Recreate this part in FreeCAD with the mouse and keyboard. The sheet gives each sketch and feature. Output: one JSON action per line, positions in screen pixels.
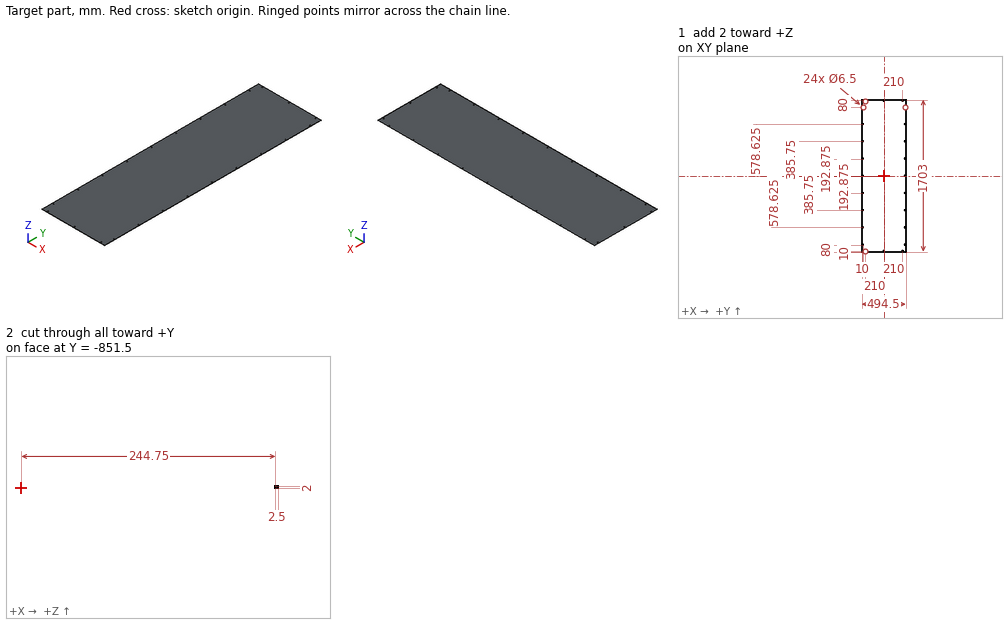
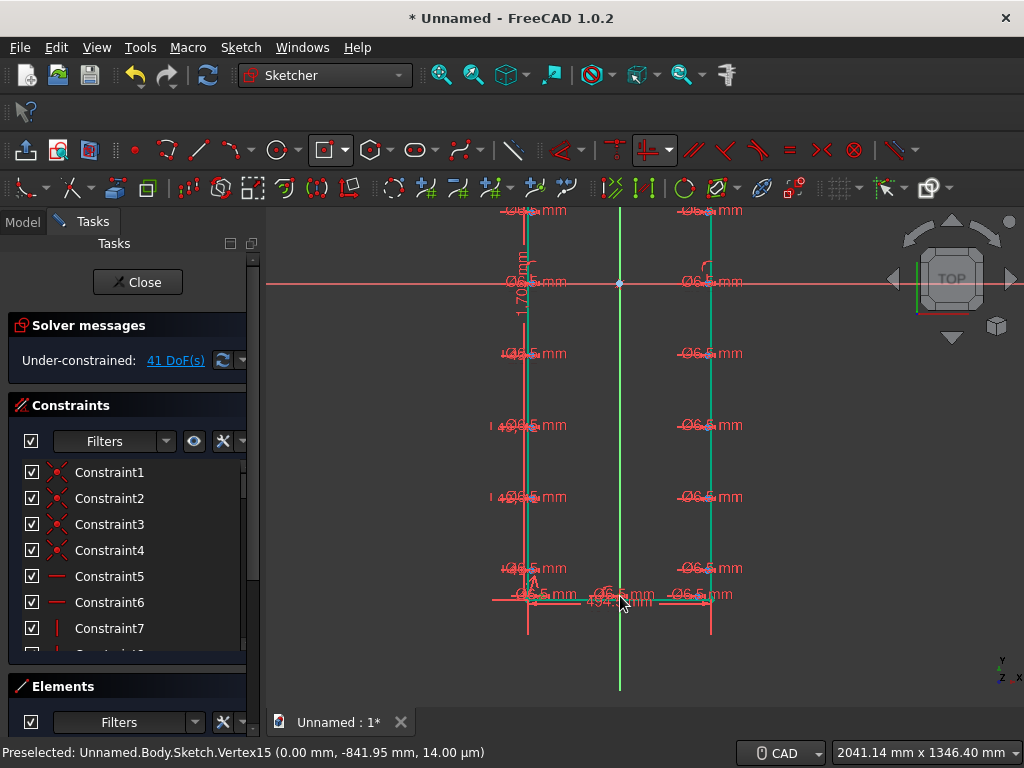
{"action": "left_click", "coordinate": [672, 150]}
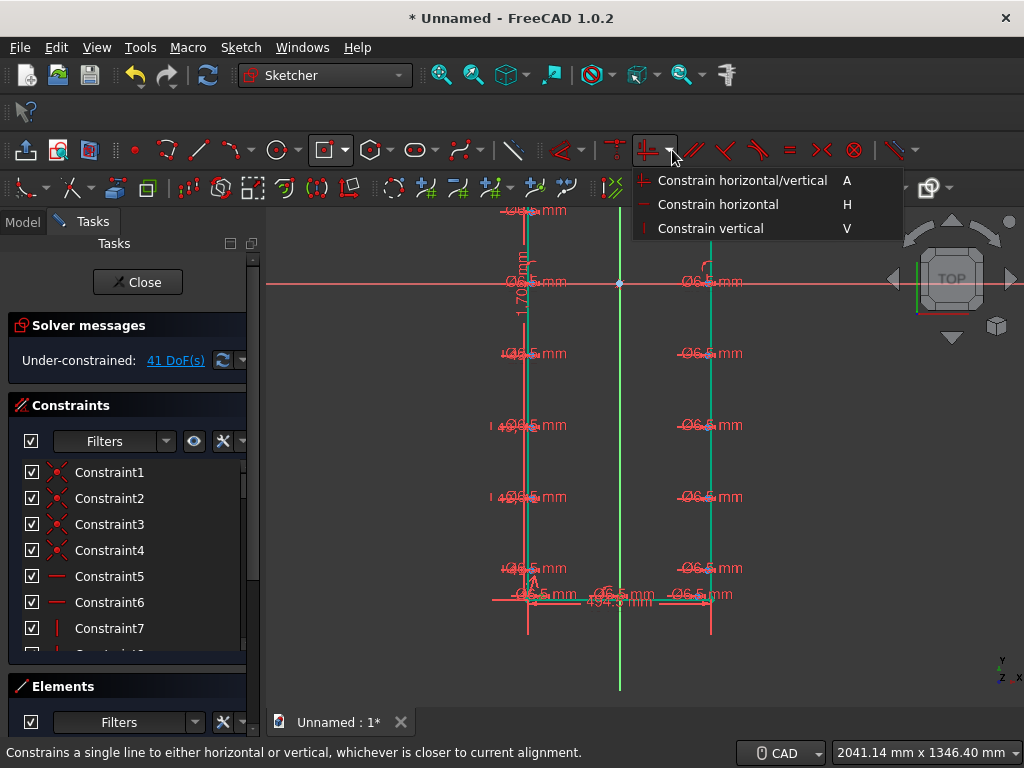
{"action": "left_click", "coordinate": [768, 204]}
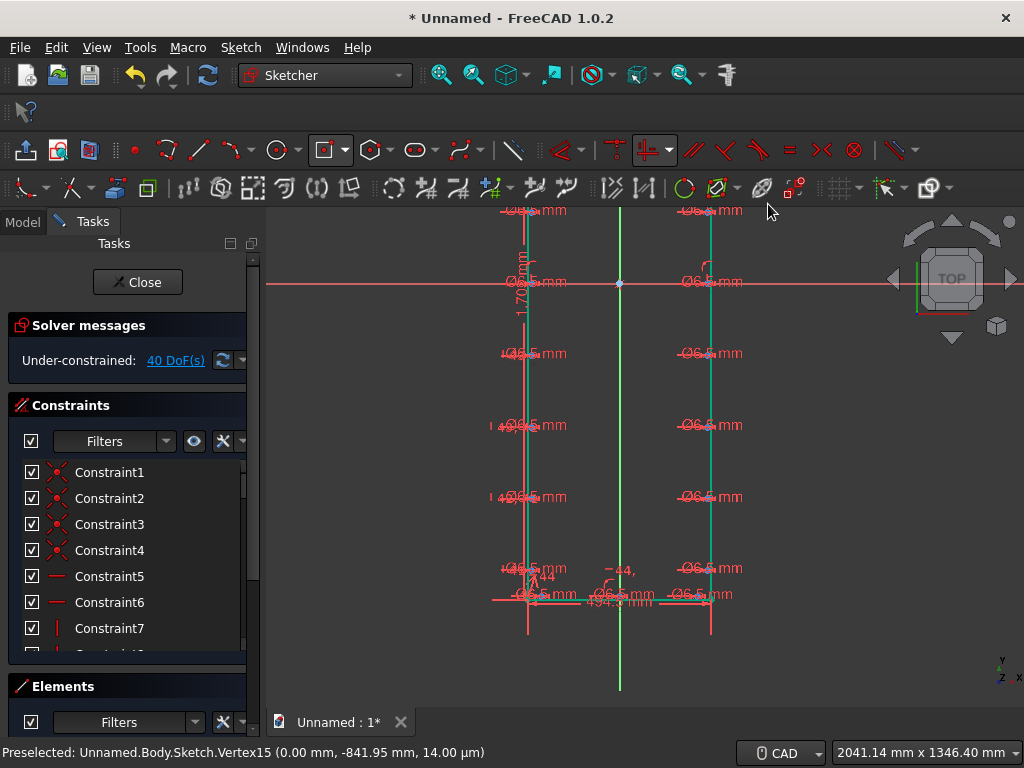
{"action": "left_click", "coordinate": [620, 596]}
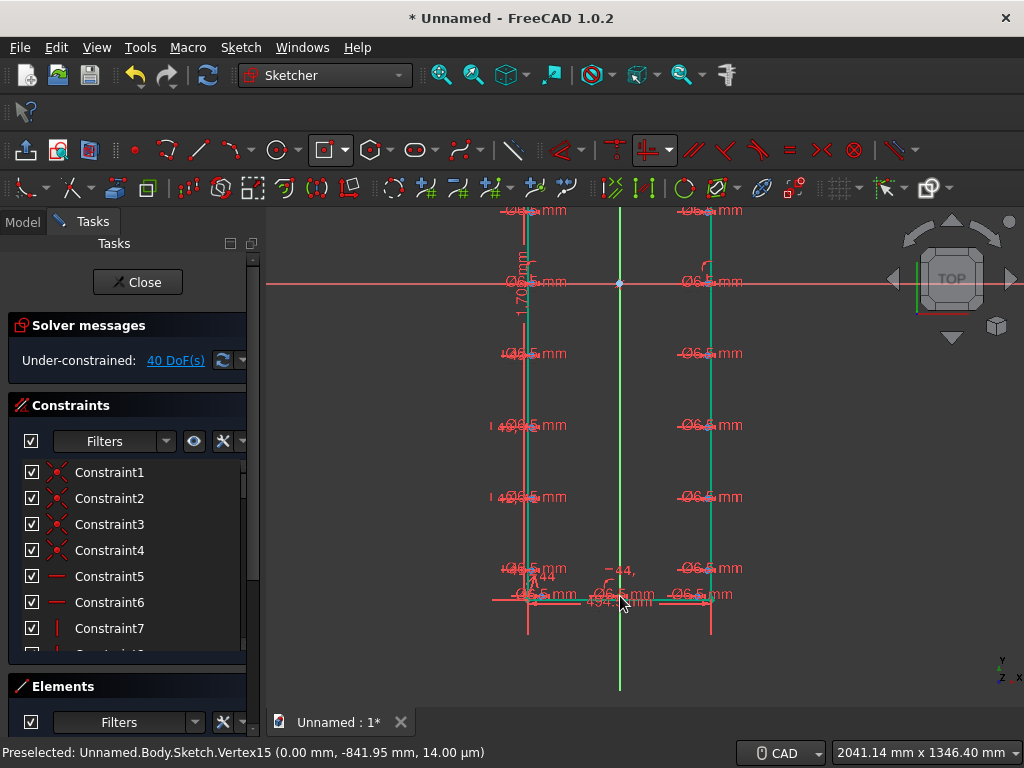
{"action": "left_click", "coordinate": [698, 596]}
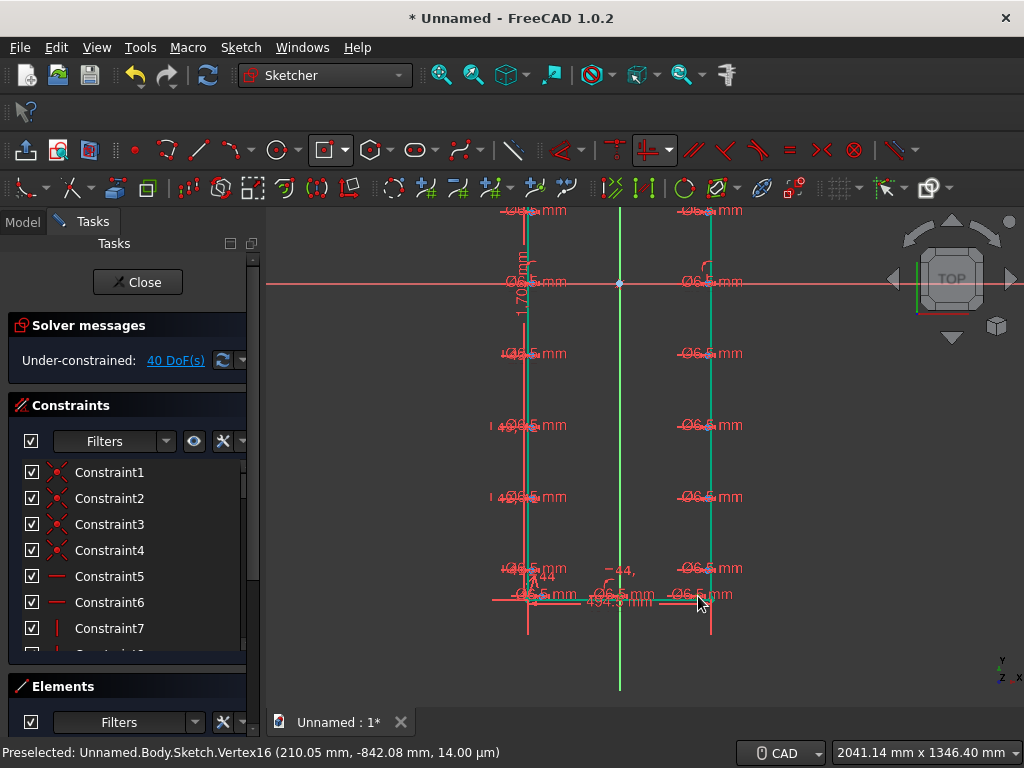
{"action": "left_click", "coordinate": [672, 150]}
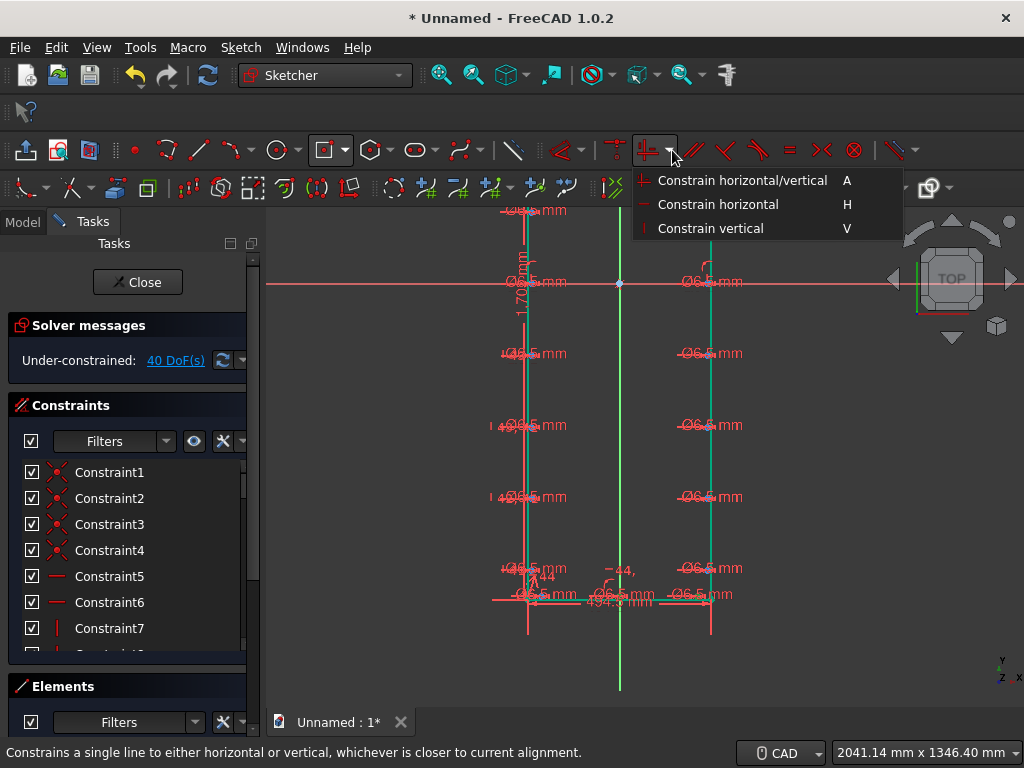
{"action": "left_click", "coordinate": [768, 204]}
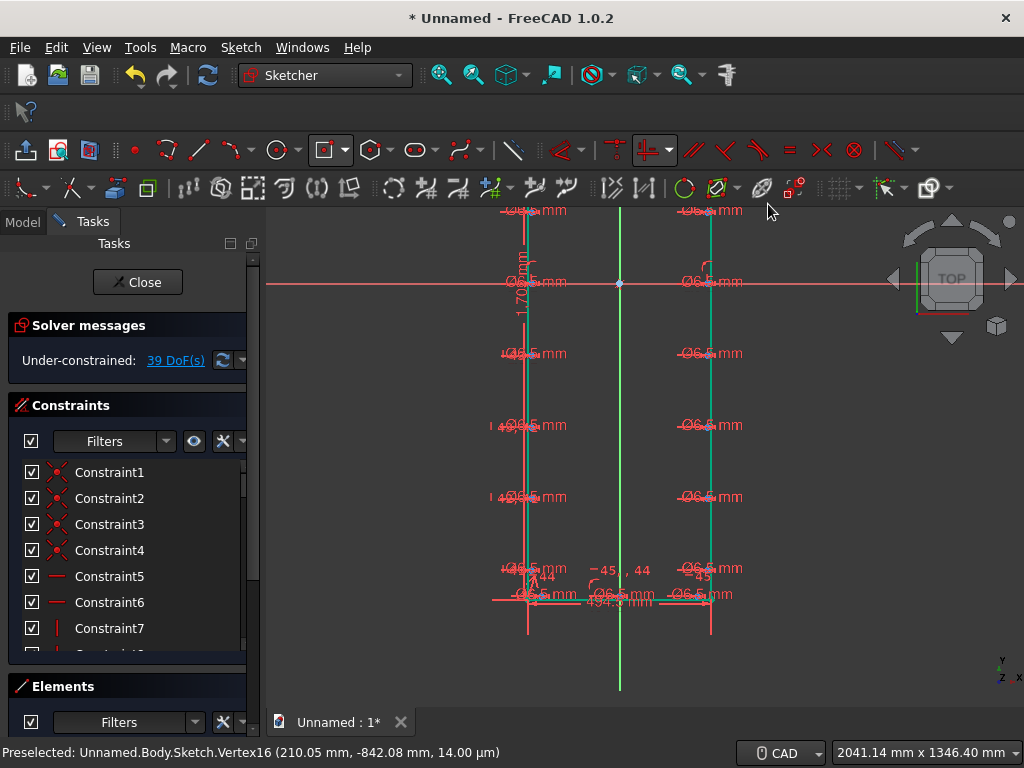
{"action": "left_click", "coordinate": [532, 570]}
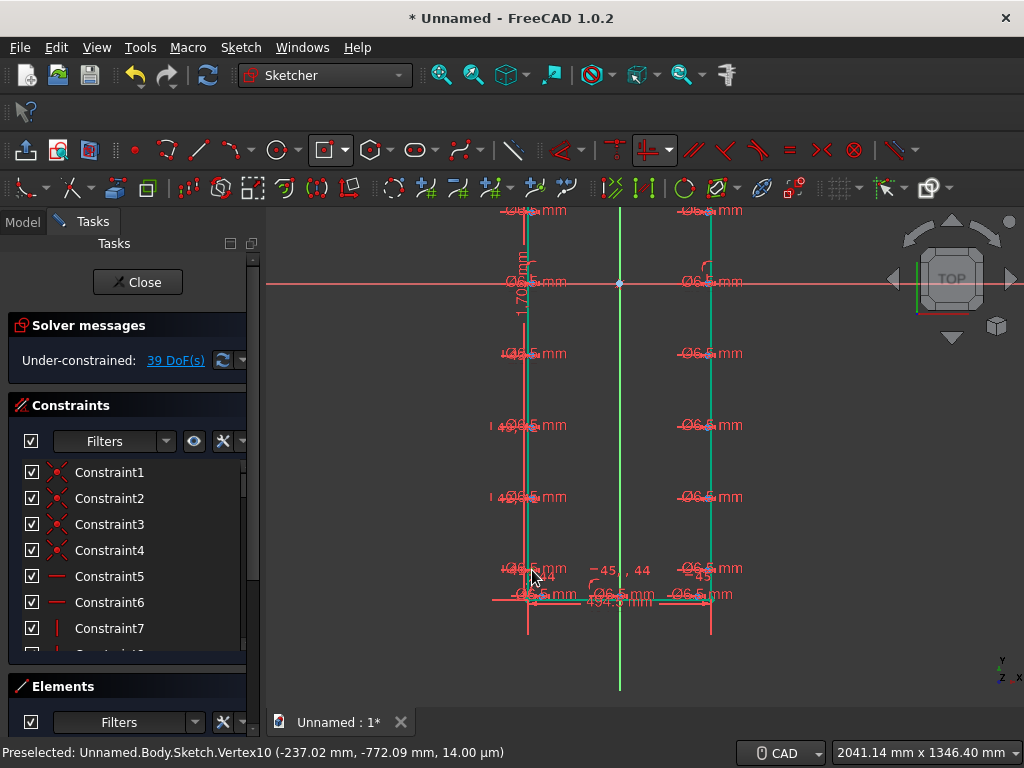
{"action": "scroll", "coordinate": [708, 570], "scroll_direction": "up", "scroll_amount": 4}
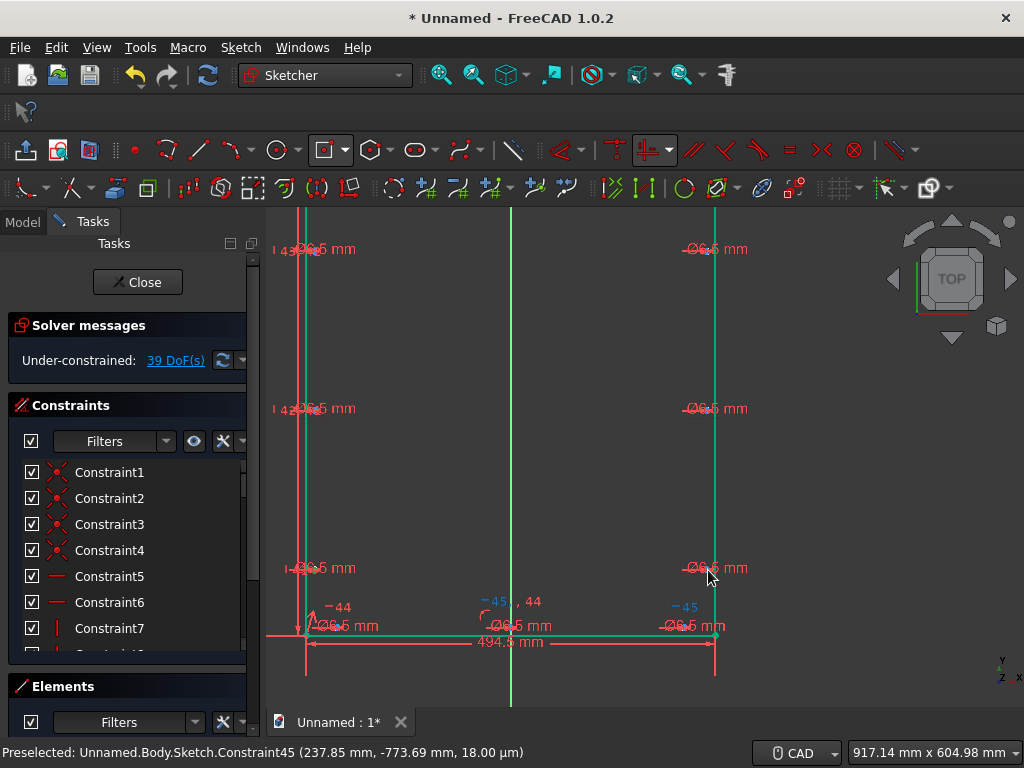
{"action": "left_click", "coordinate": [707, 570]}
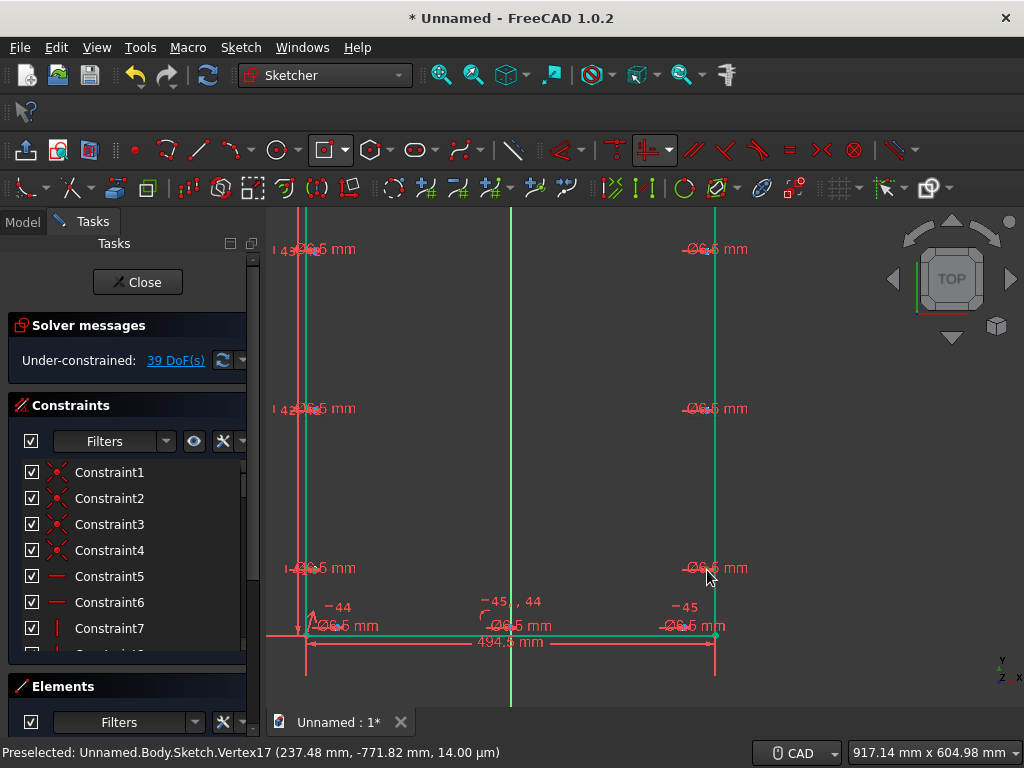
{"action": "key", "text": "h"}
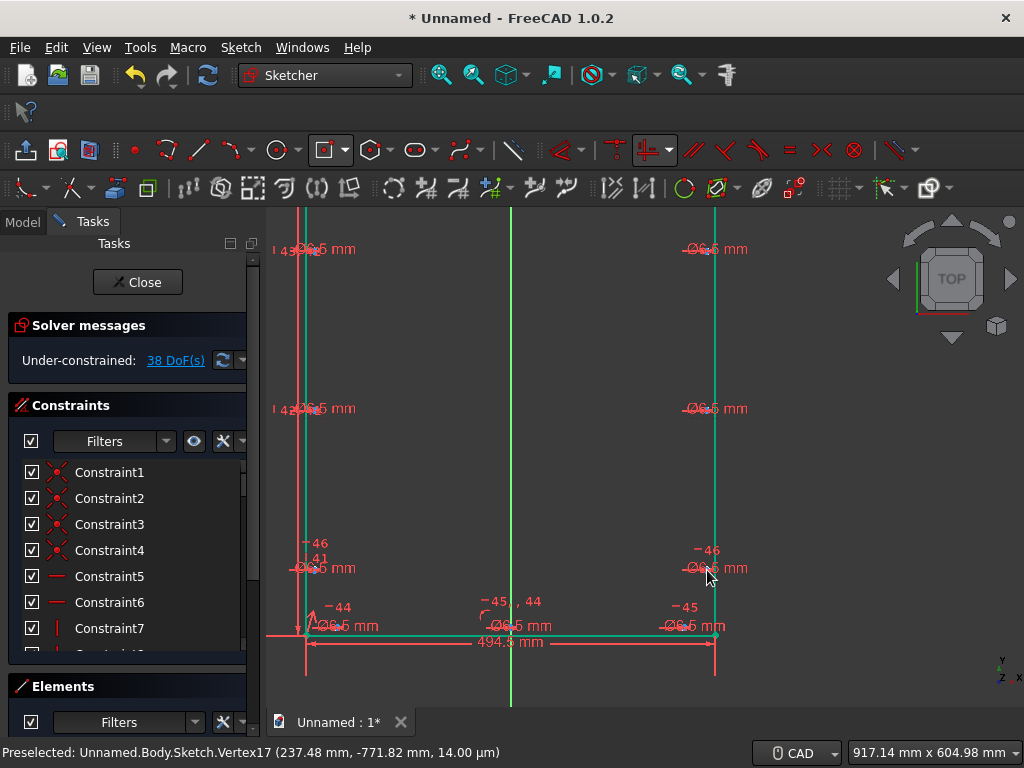
{"action": "scroll", "coordinate": [593, 590], "scroll_direction": "down", "scroll_amount": 8}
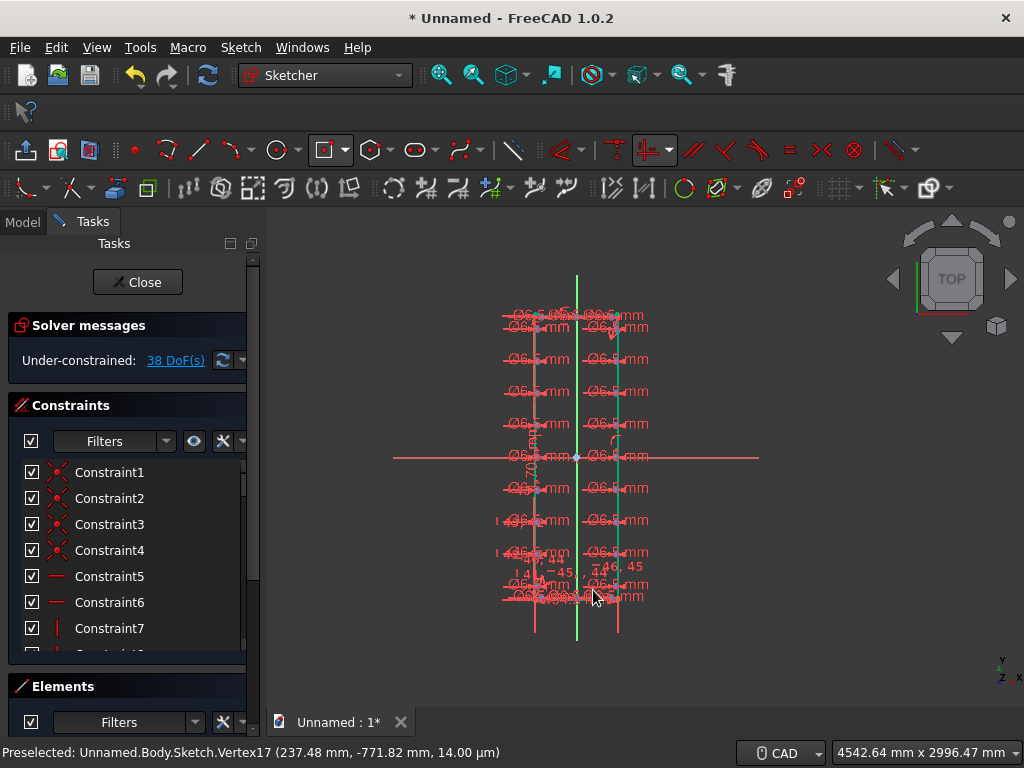
{"action": "left_click", "coordinate": [616, 587]}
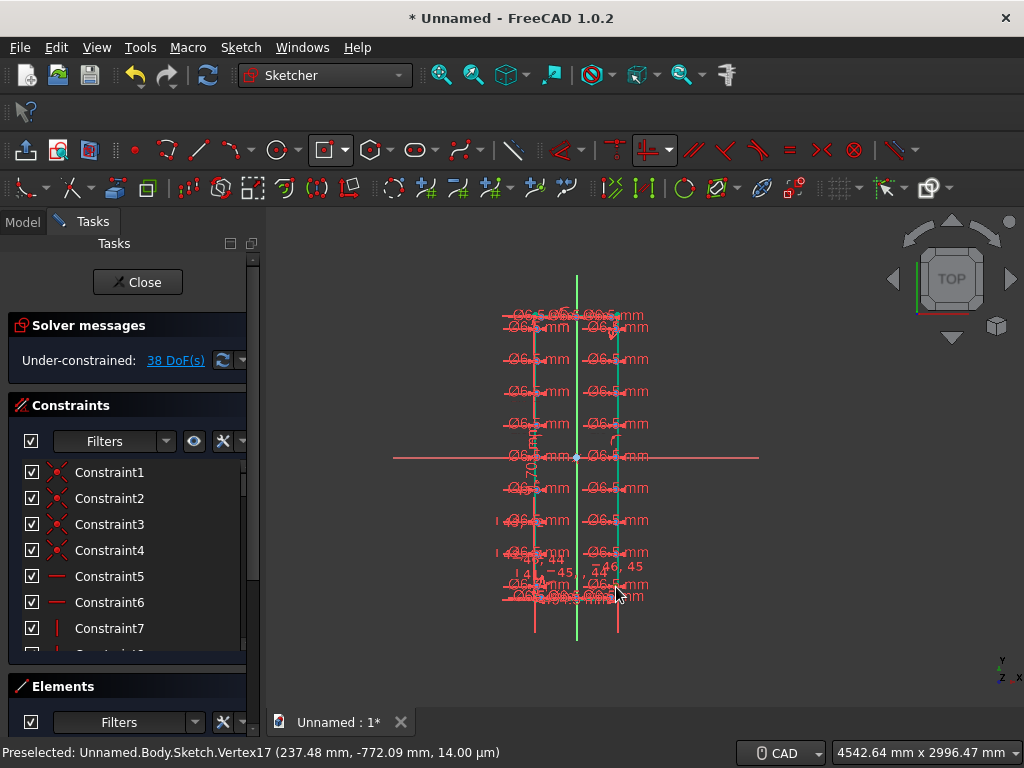
{"action": "left_click", "coordinate": [616, 554]}